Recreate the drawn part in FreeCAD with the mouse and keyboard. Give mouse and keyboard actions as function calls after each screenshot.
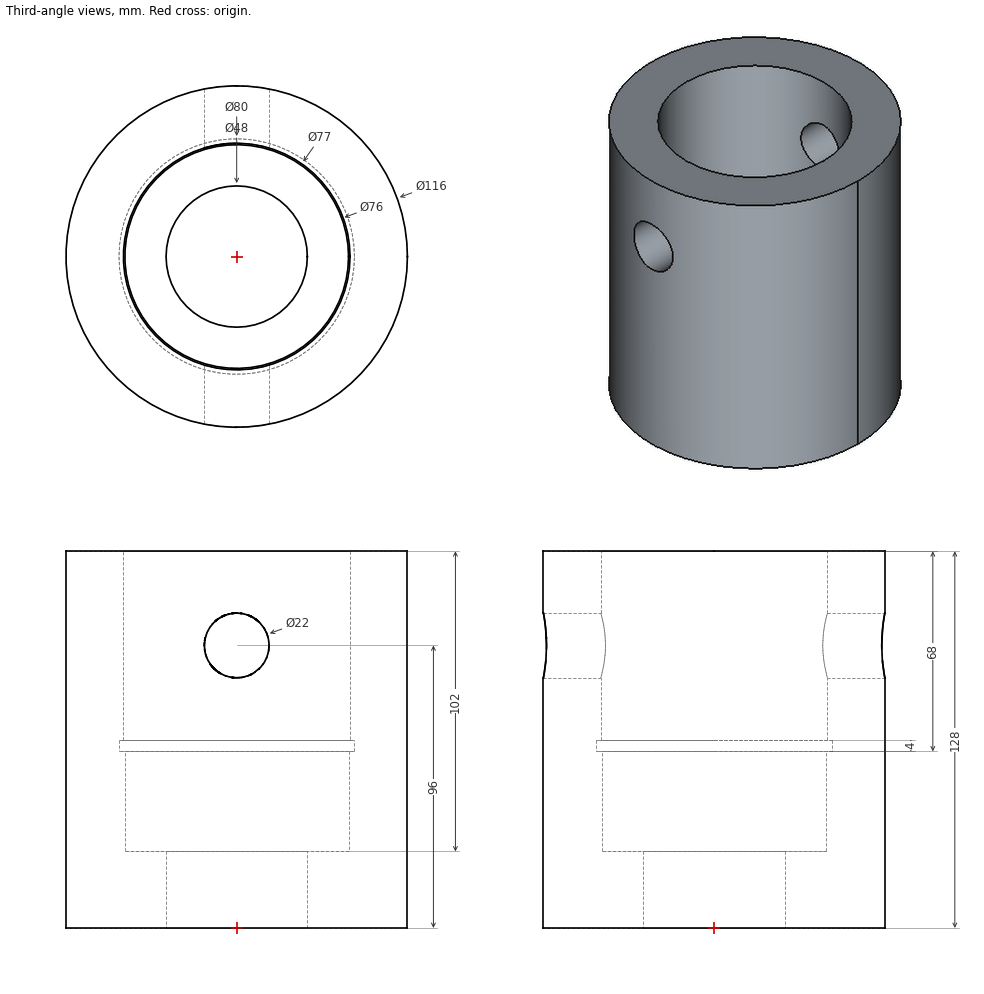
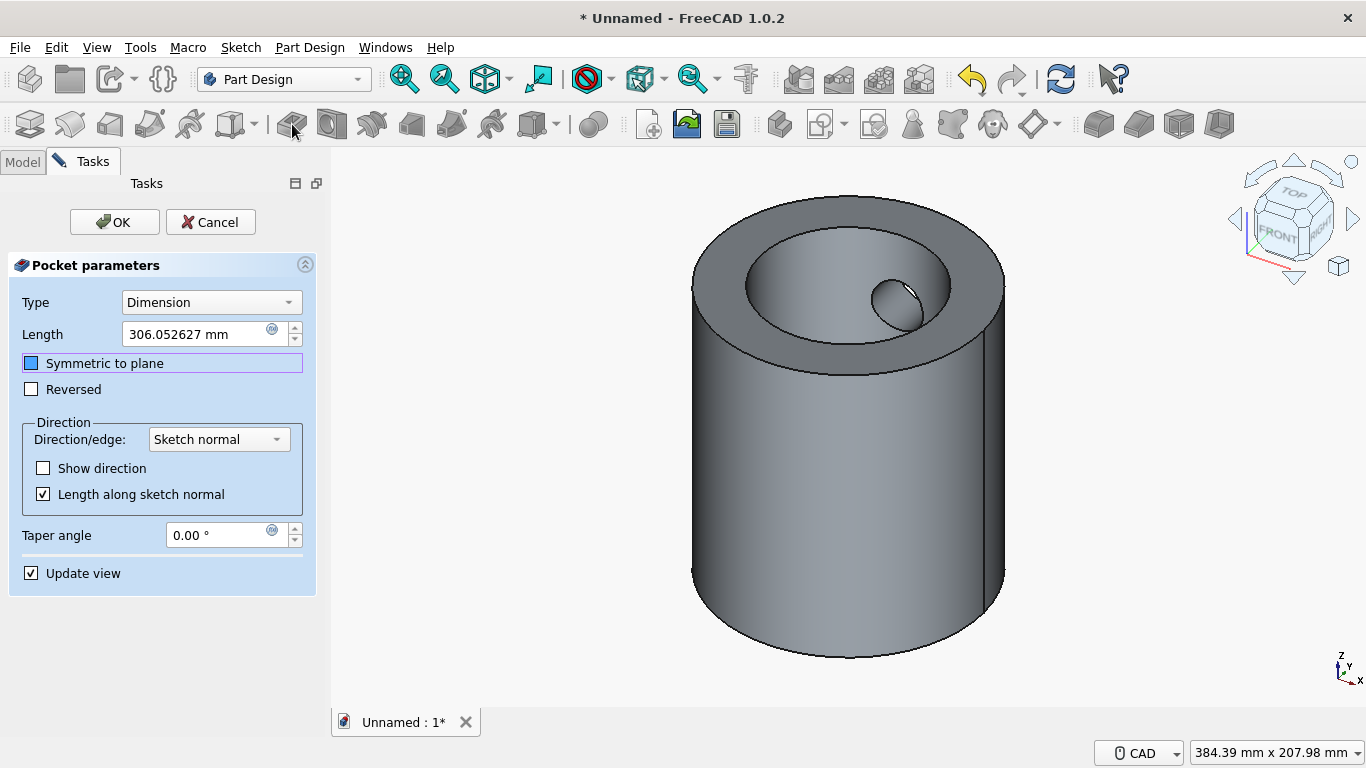
click(30, 363)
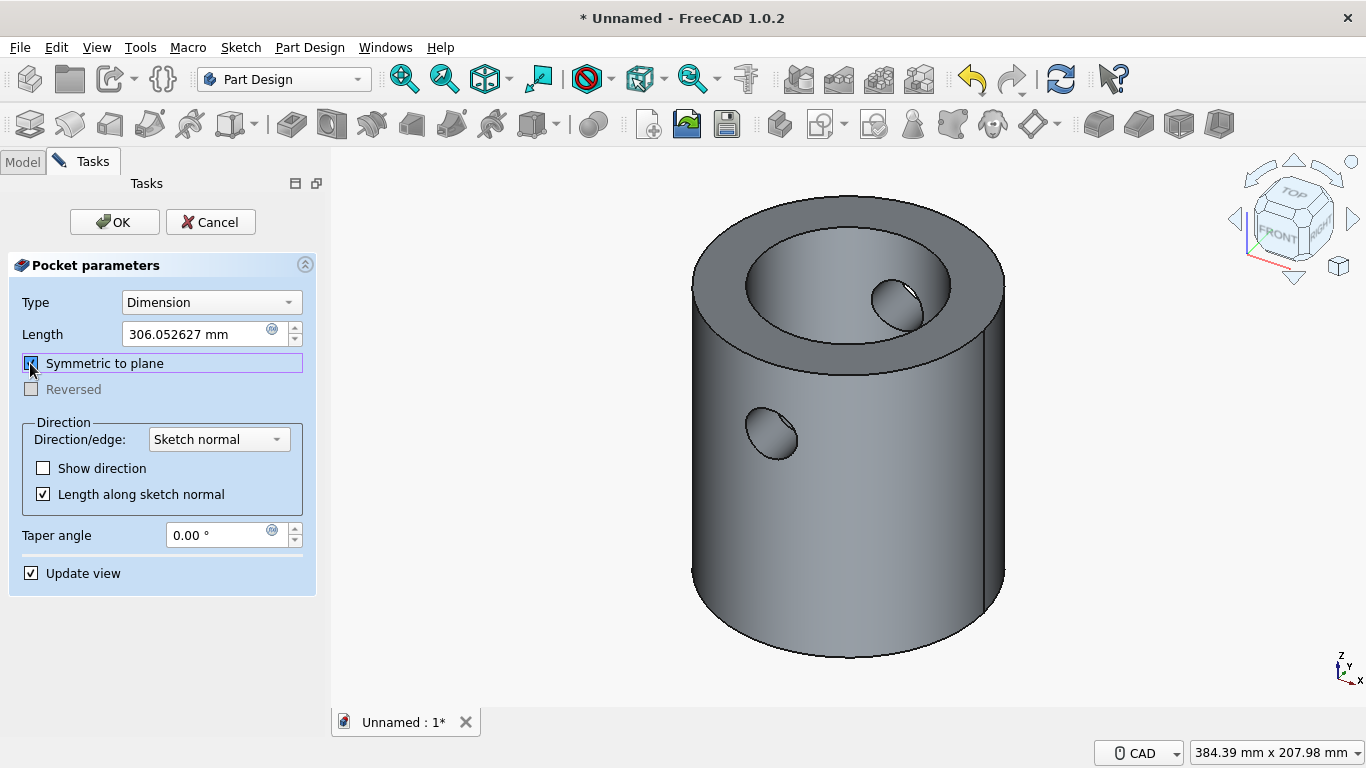
click(115, 222)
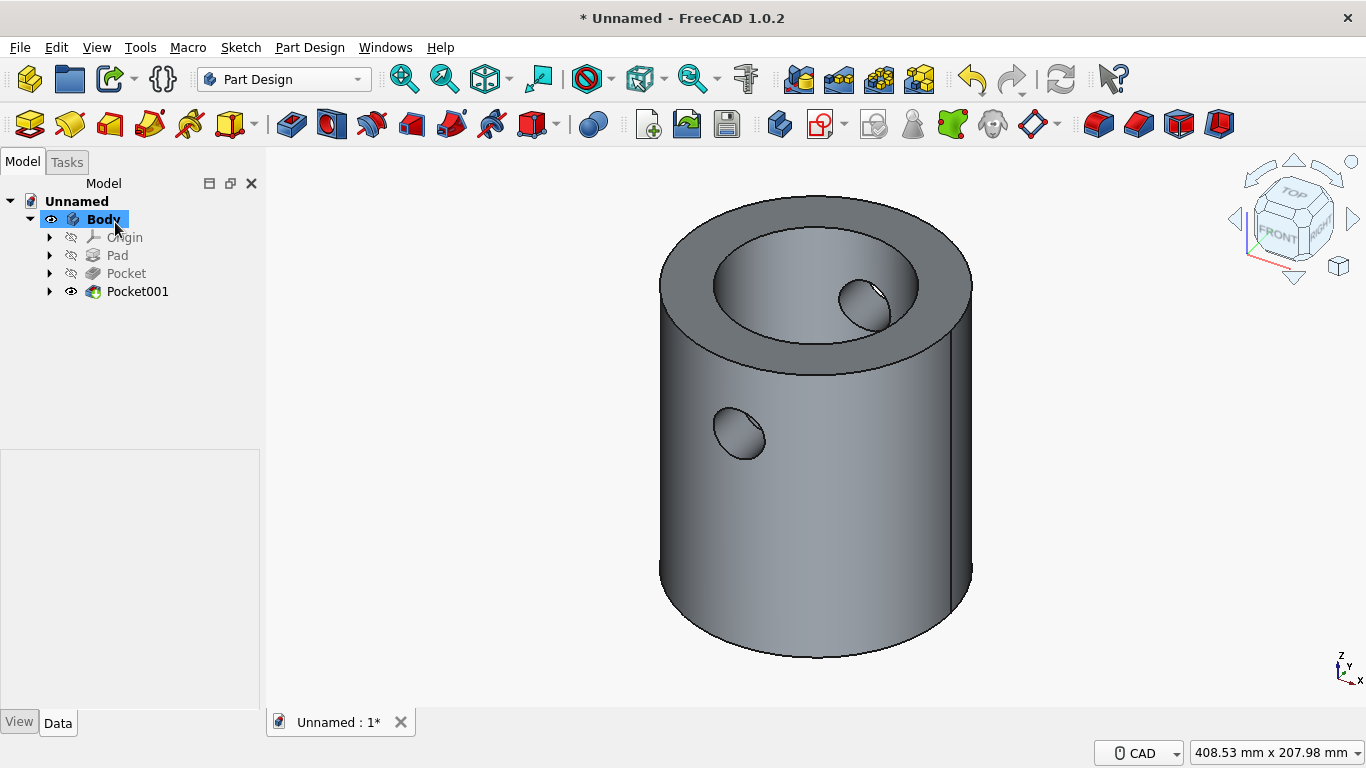
click(938, 266)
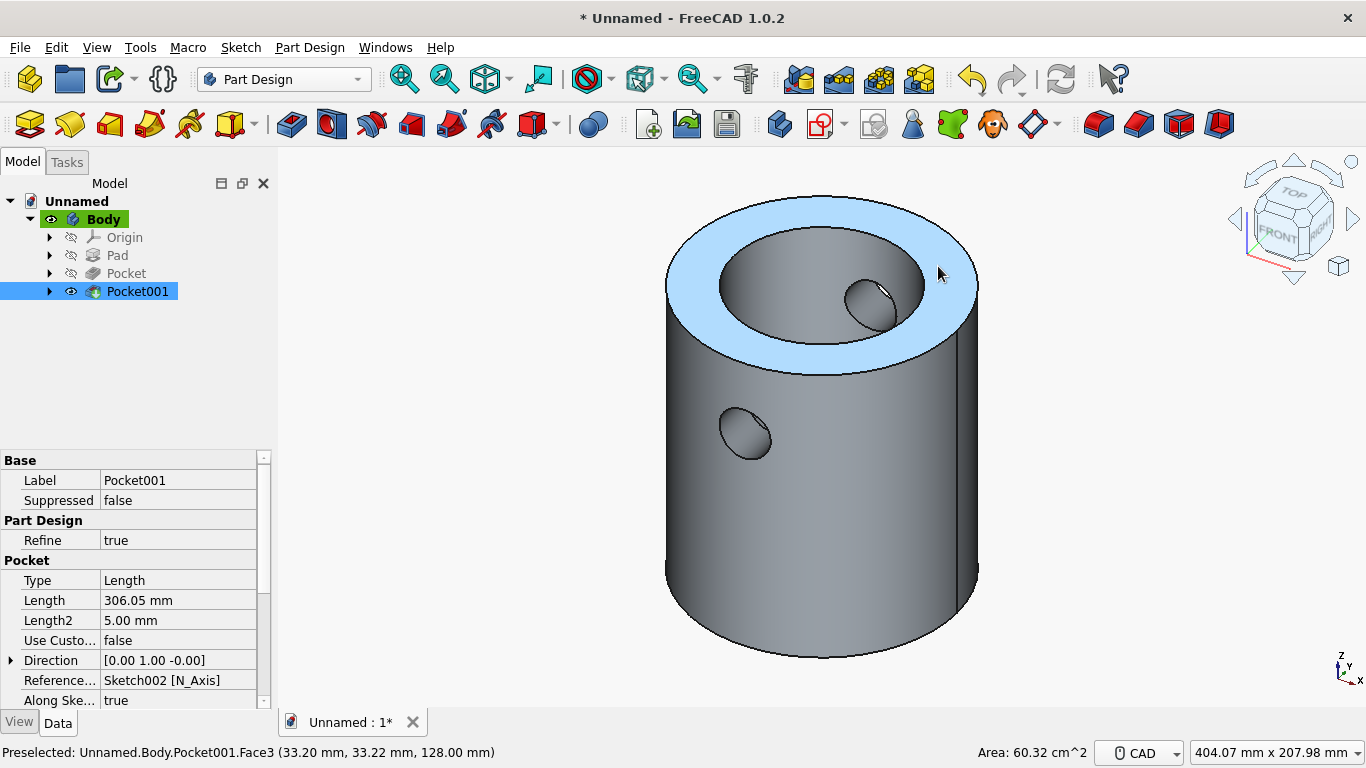
click(820, 124)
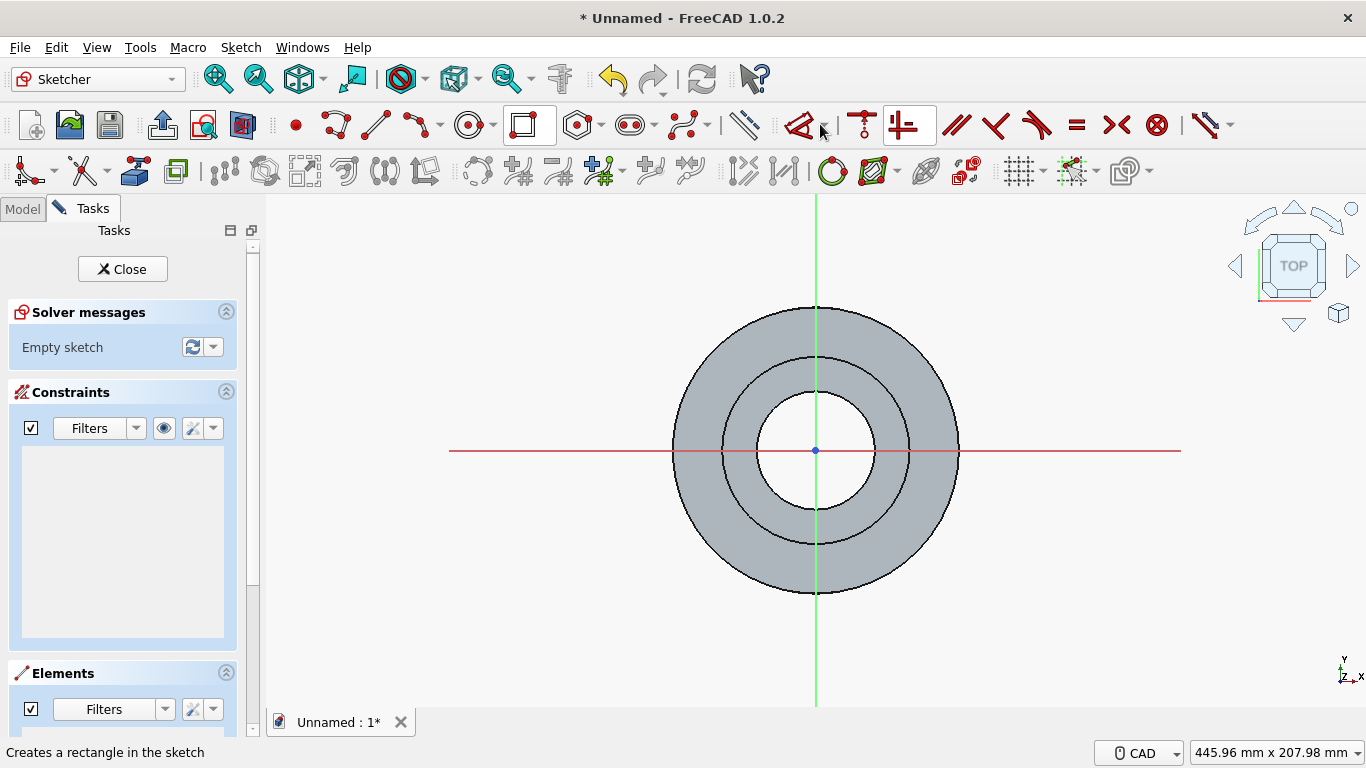
scroll(899, 450, up, 3)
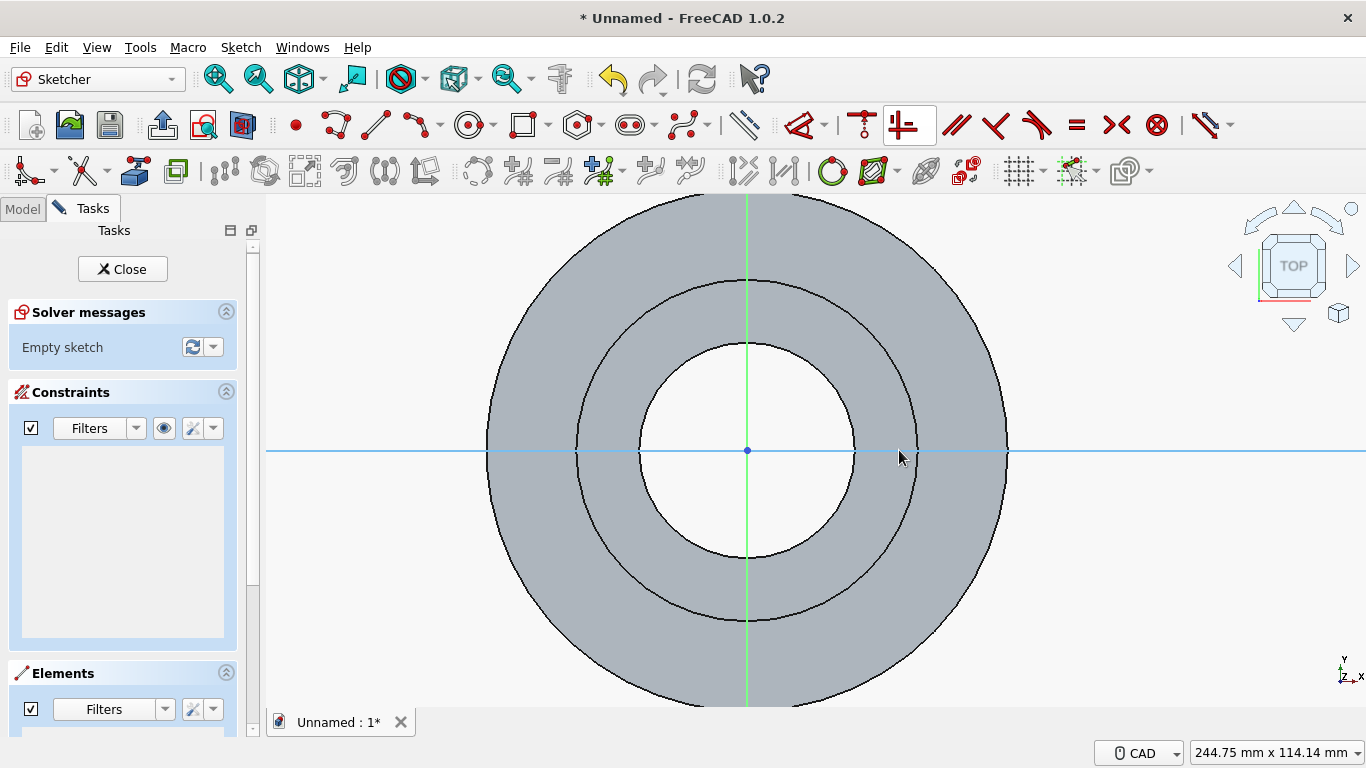
click(470, 126)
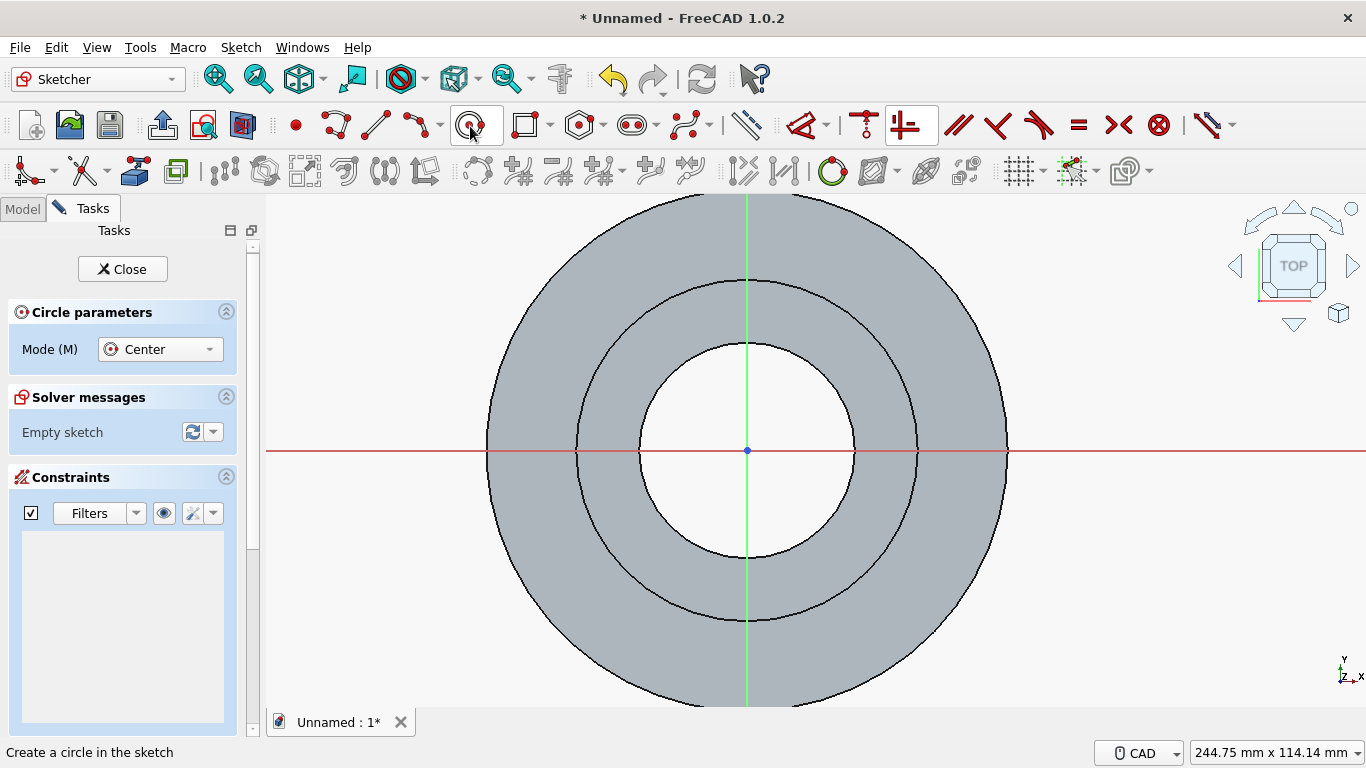
click(747, 450)
move(869, 328)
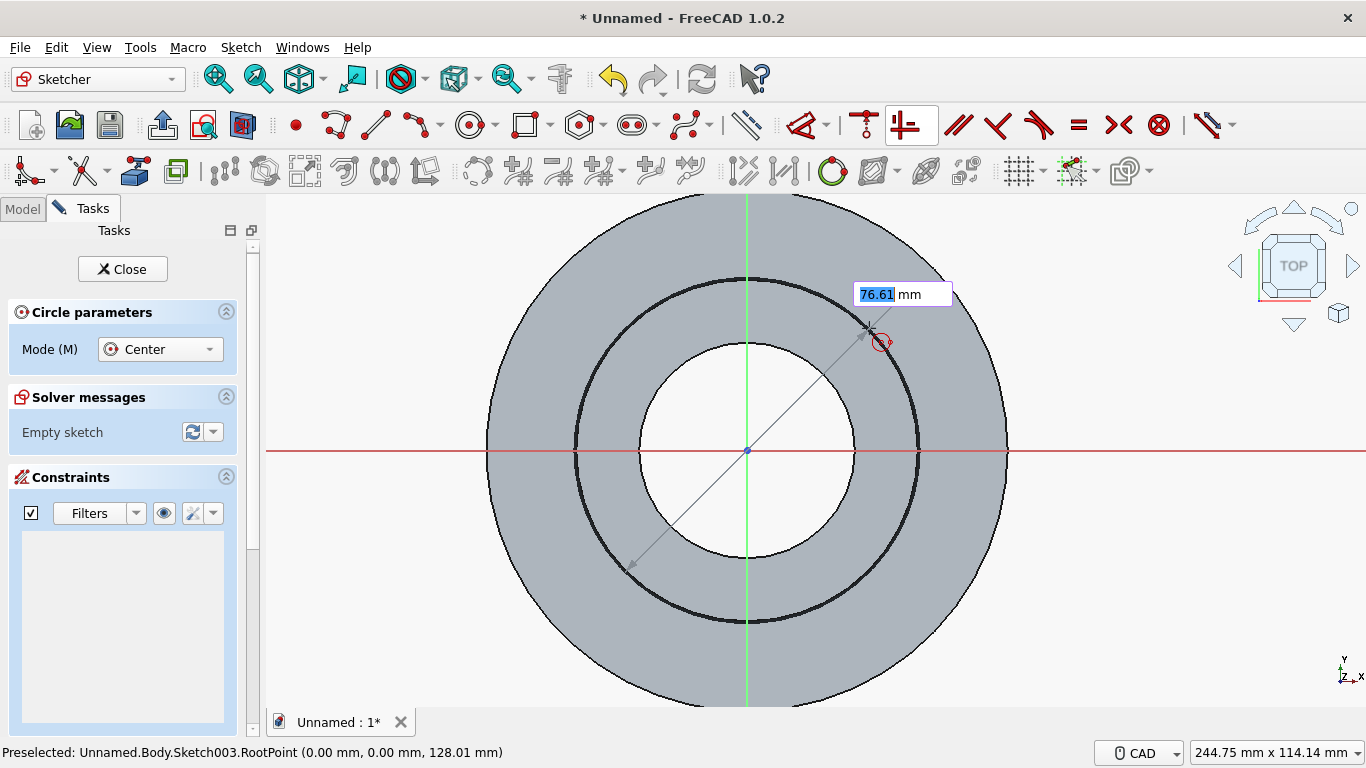
text(77)
key(Return)
key(Escape)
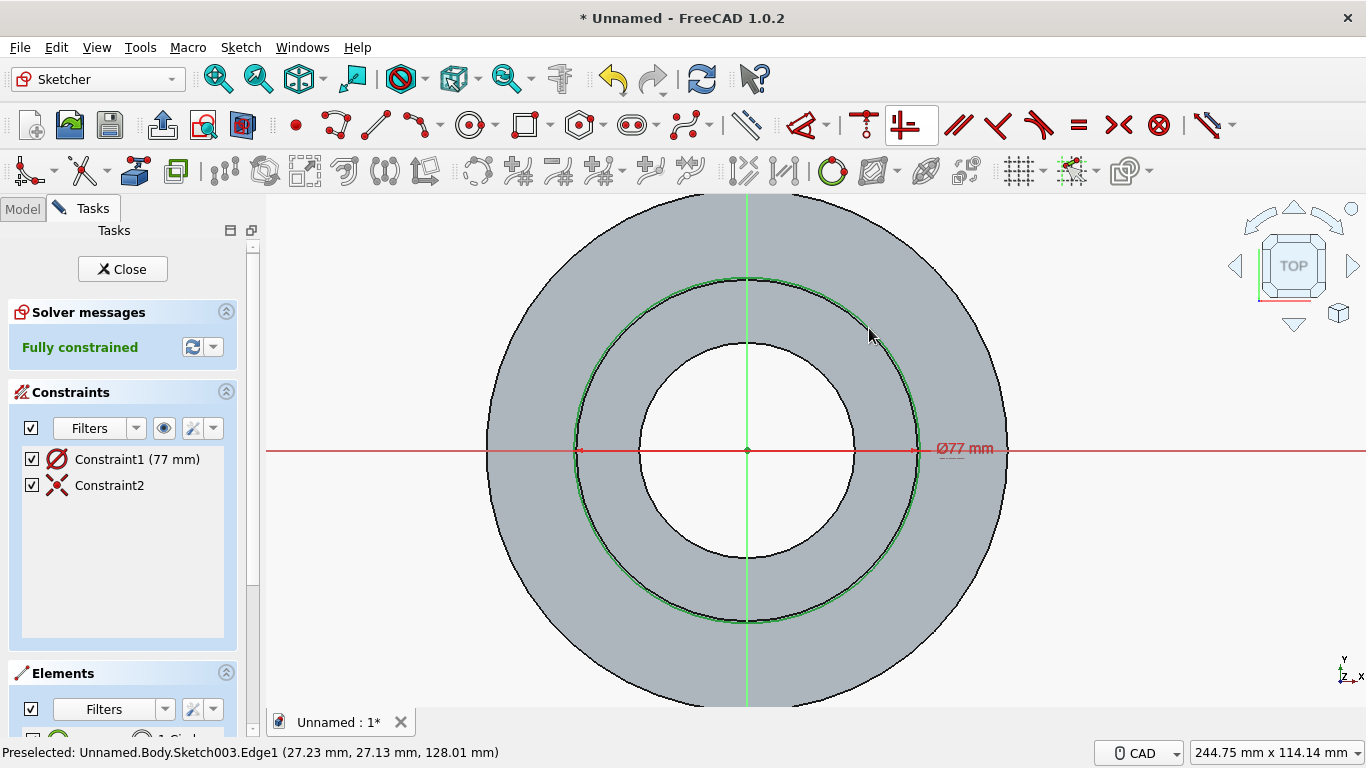
click(123, 269)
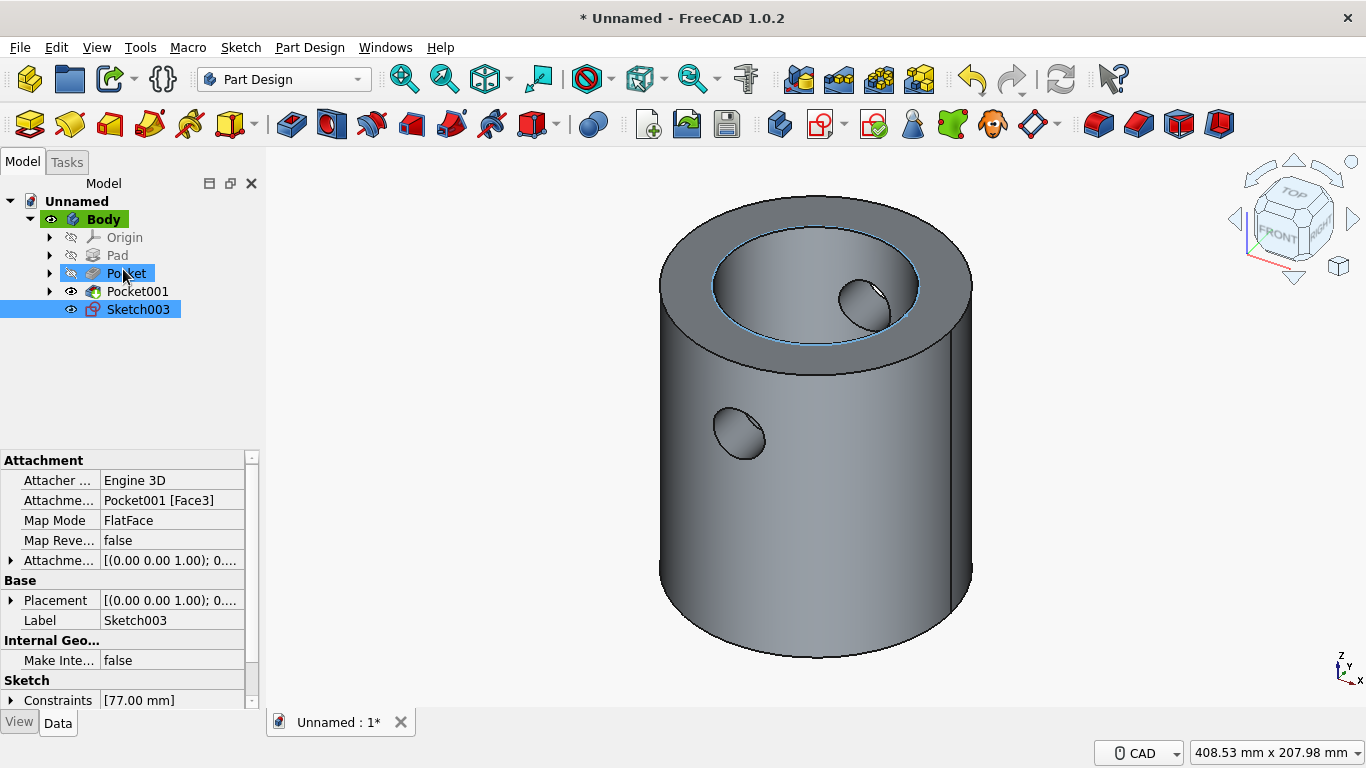
click(292, 124)